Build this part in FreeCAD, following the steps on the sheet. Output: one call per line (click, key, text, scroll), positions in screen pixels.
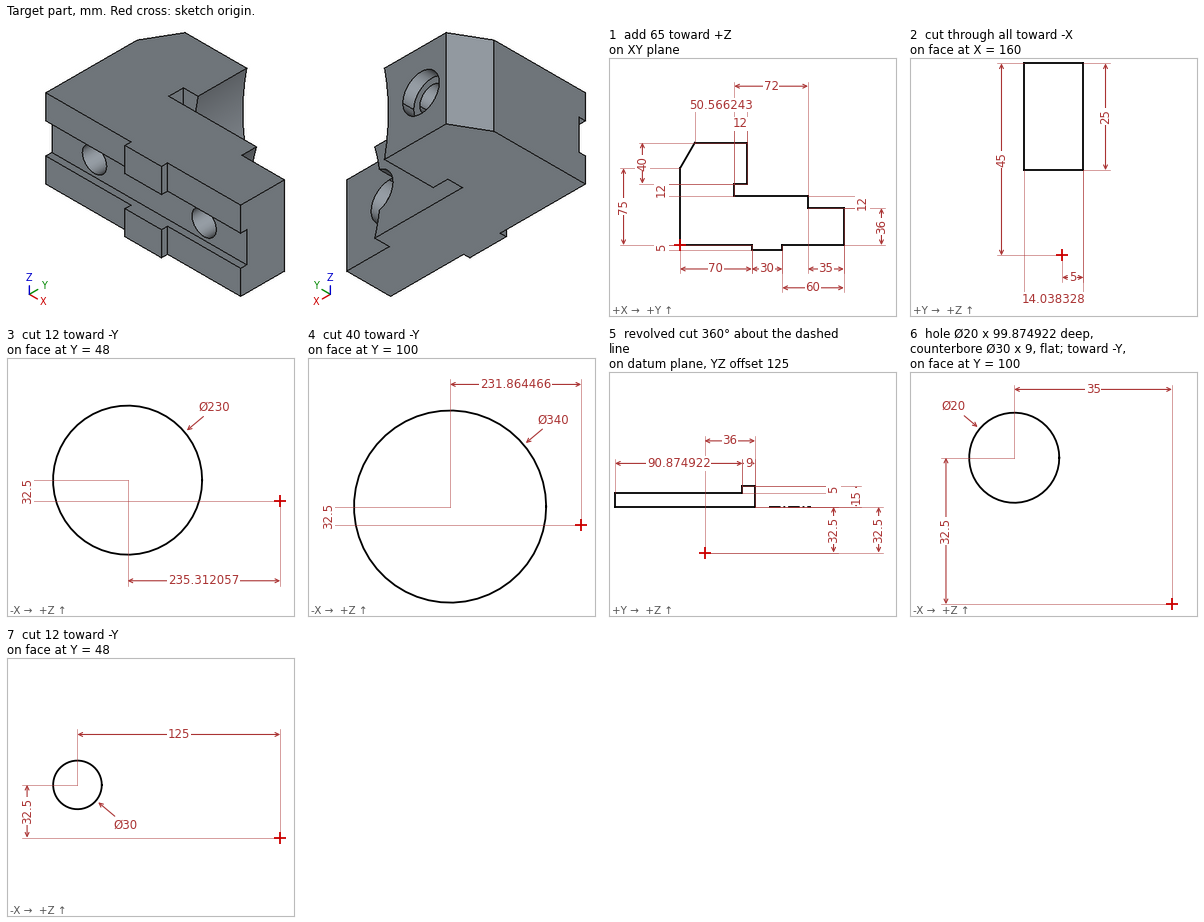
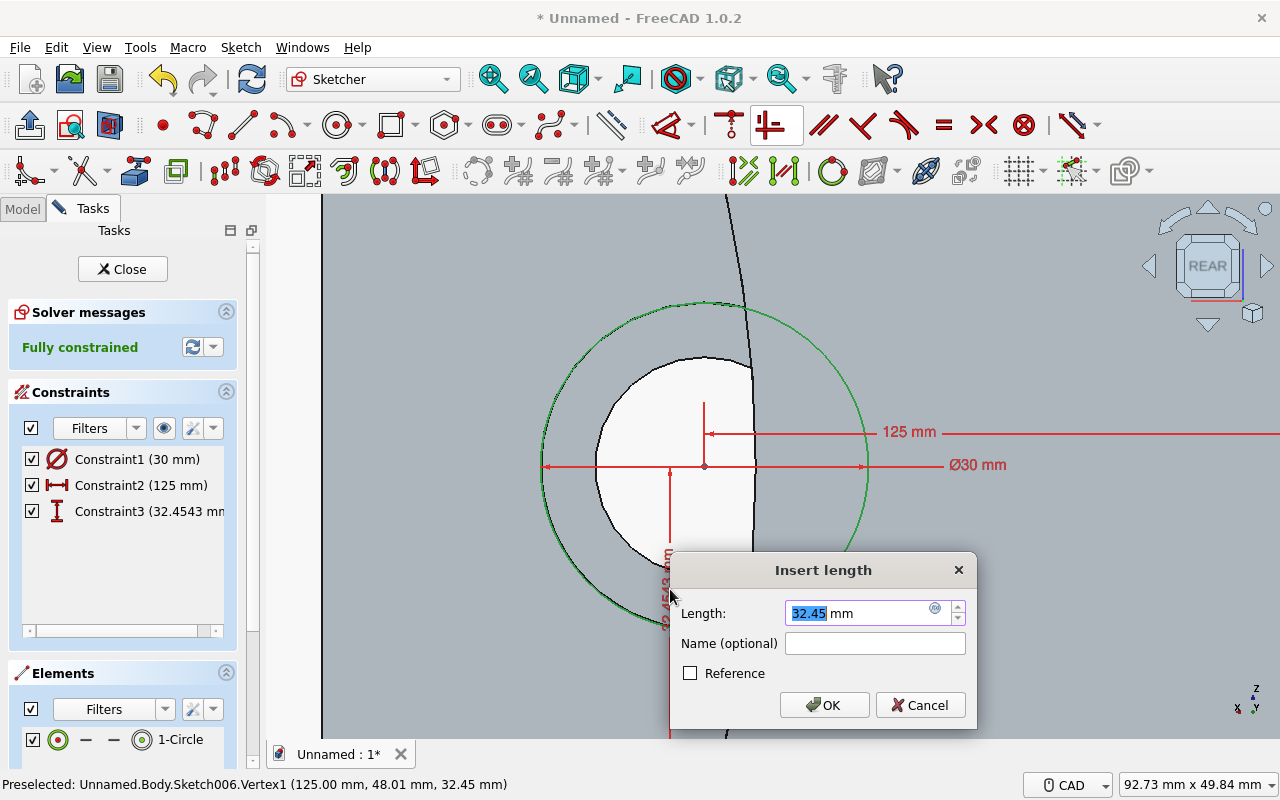
text(32.5)
key(Return)
key(Escape)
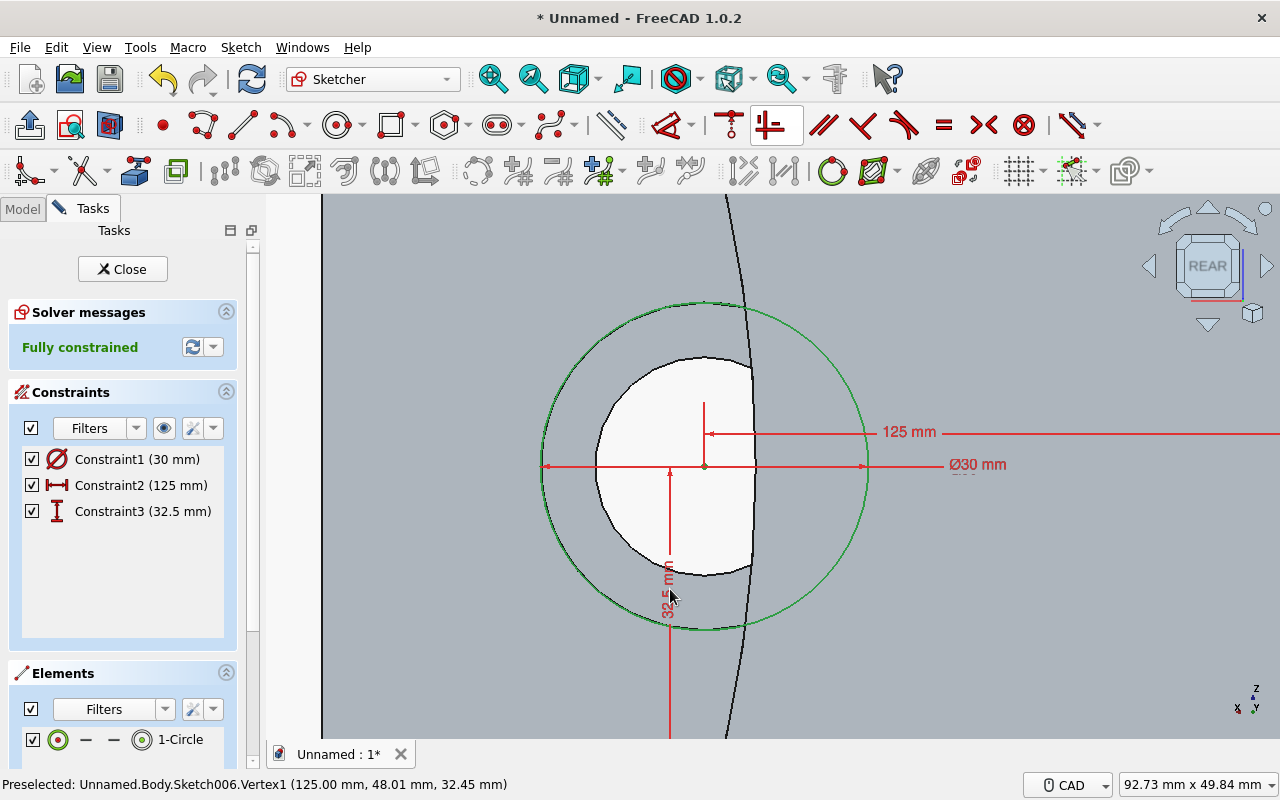
click(123, 269)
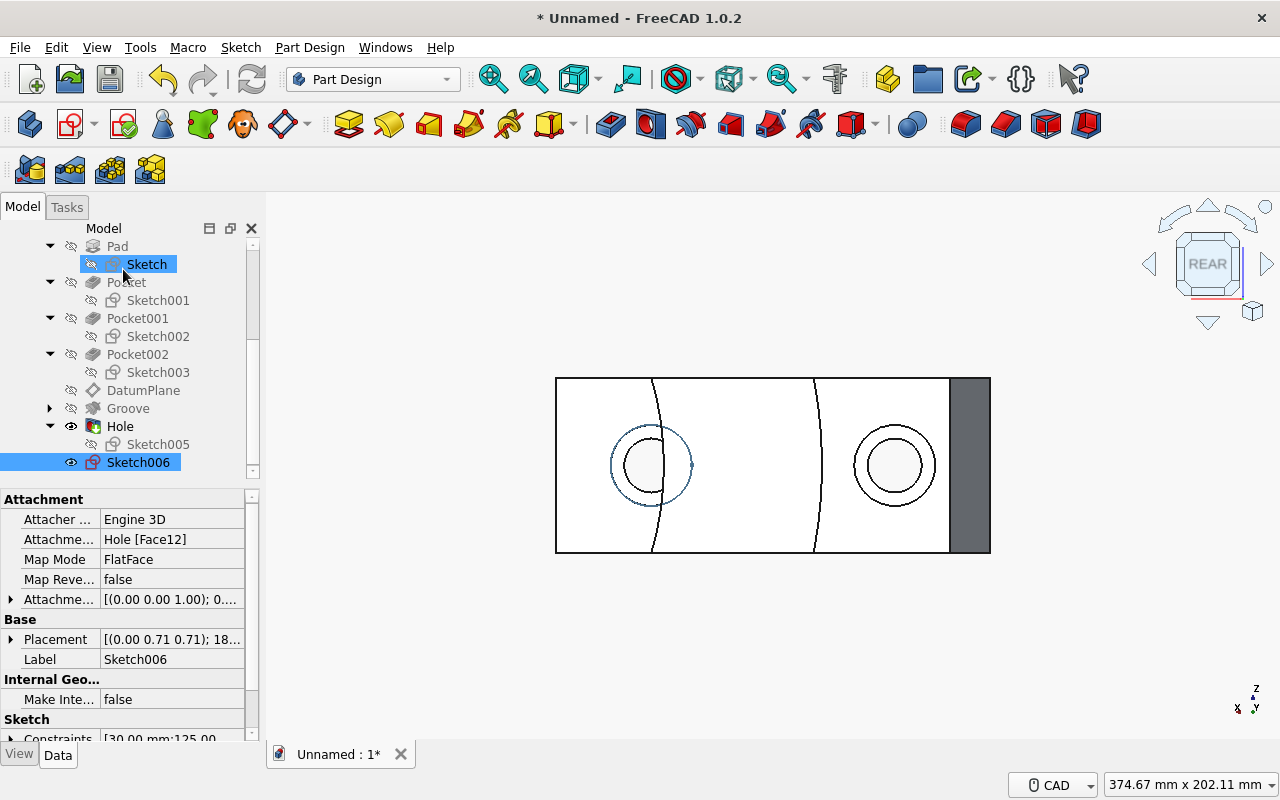
click(612, 124)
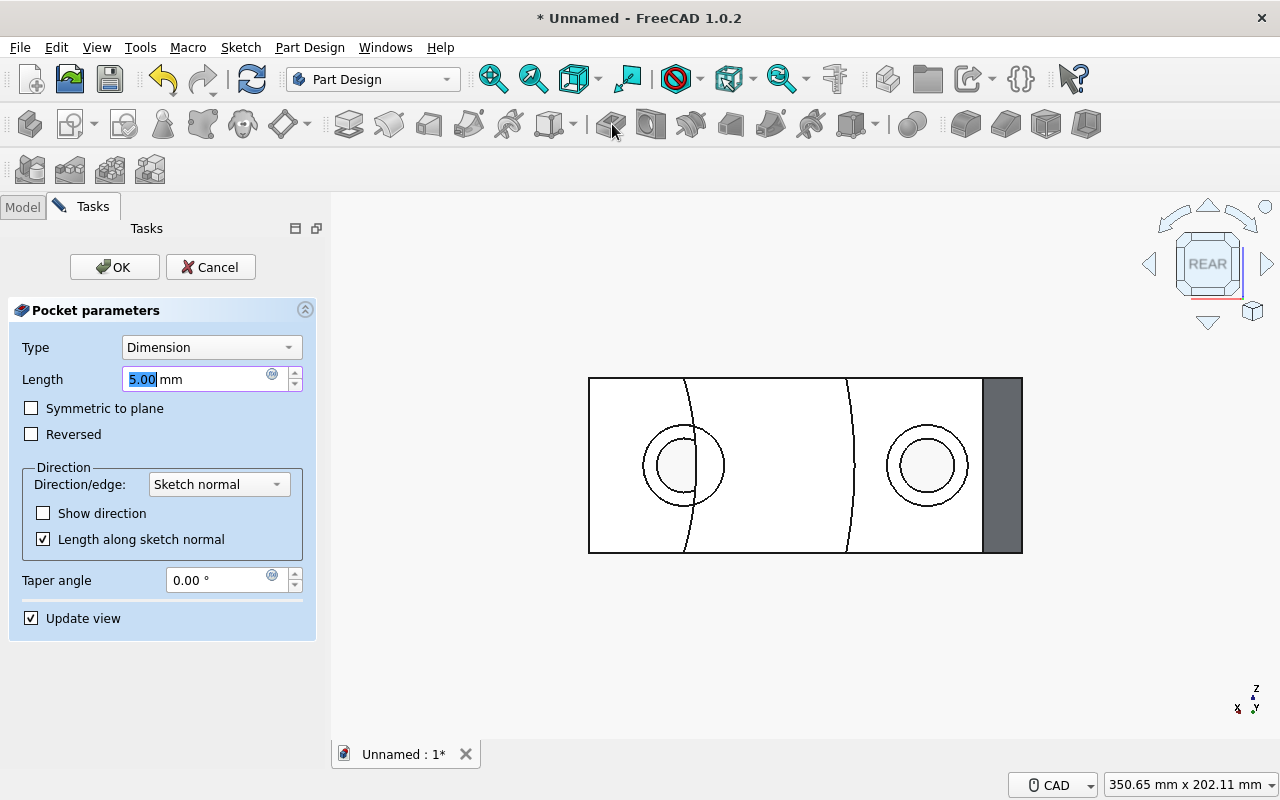
text(12)
key(Tab)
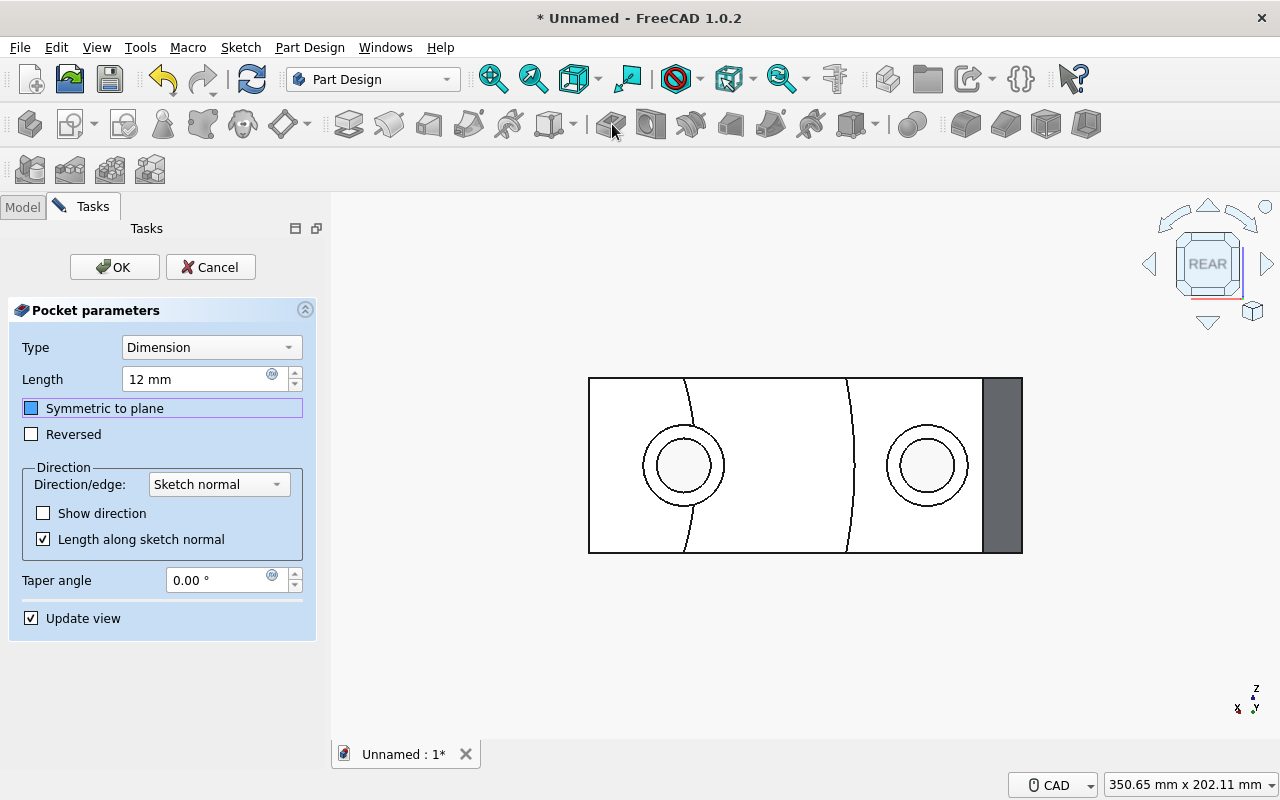
click(115, 267)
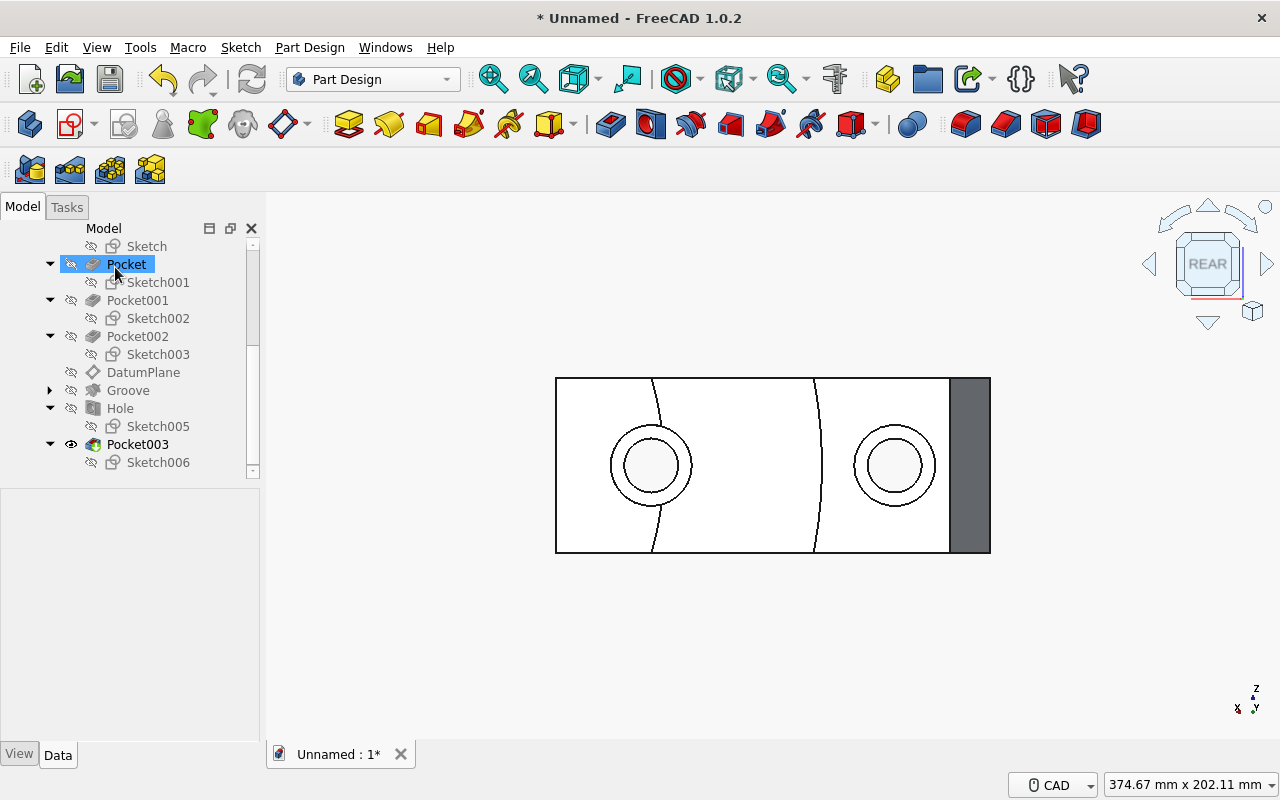
key(0)